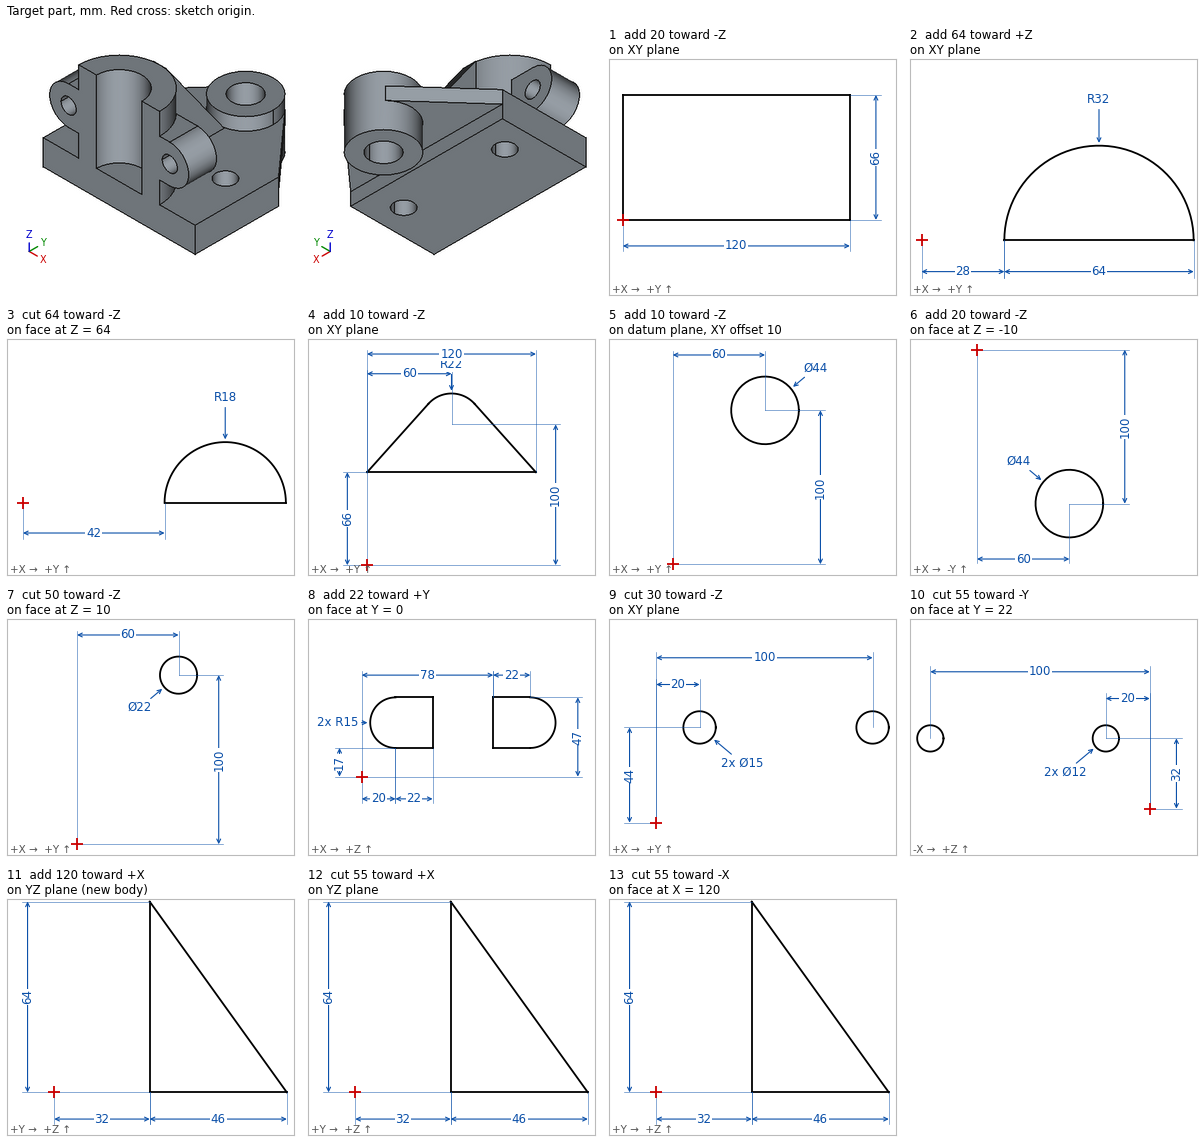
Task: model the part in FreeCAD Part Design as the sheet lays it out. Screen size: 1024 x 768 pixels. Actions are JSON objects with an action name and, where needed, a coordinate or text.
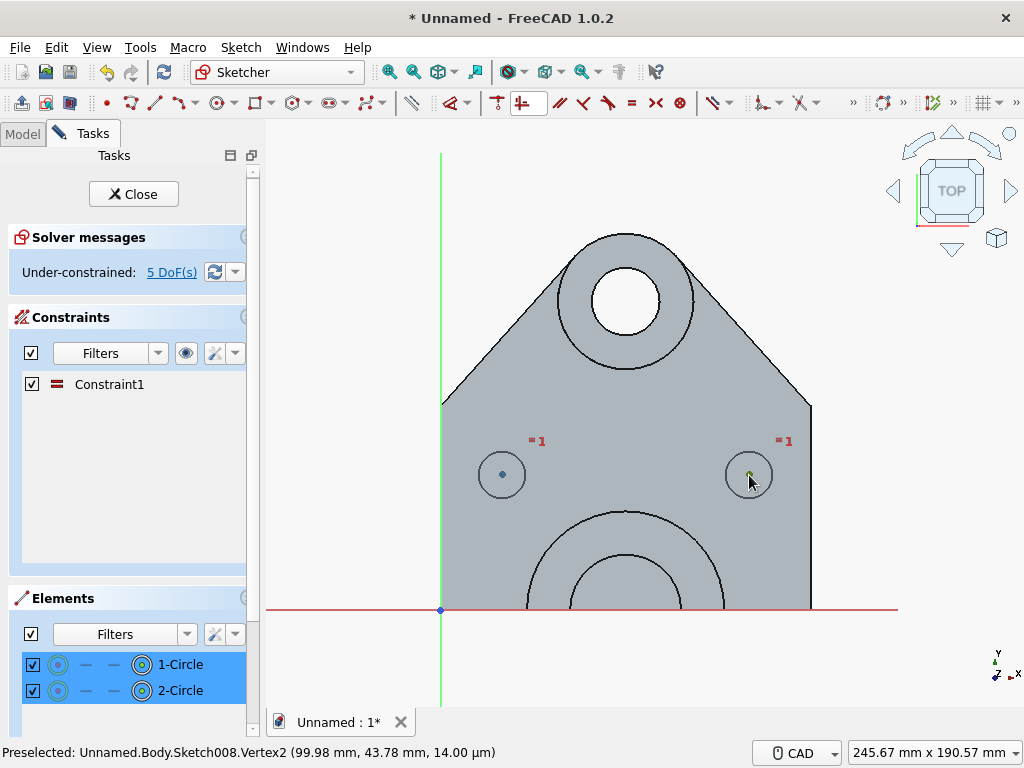
{"action": "key", "text": "h"}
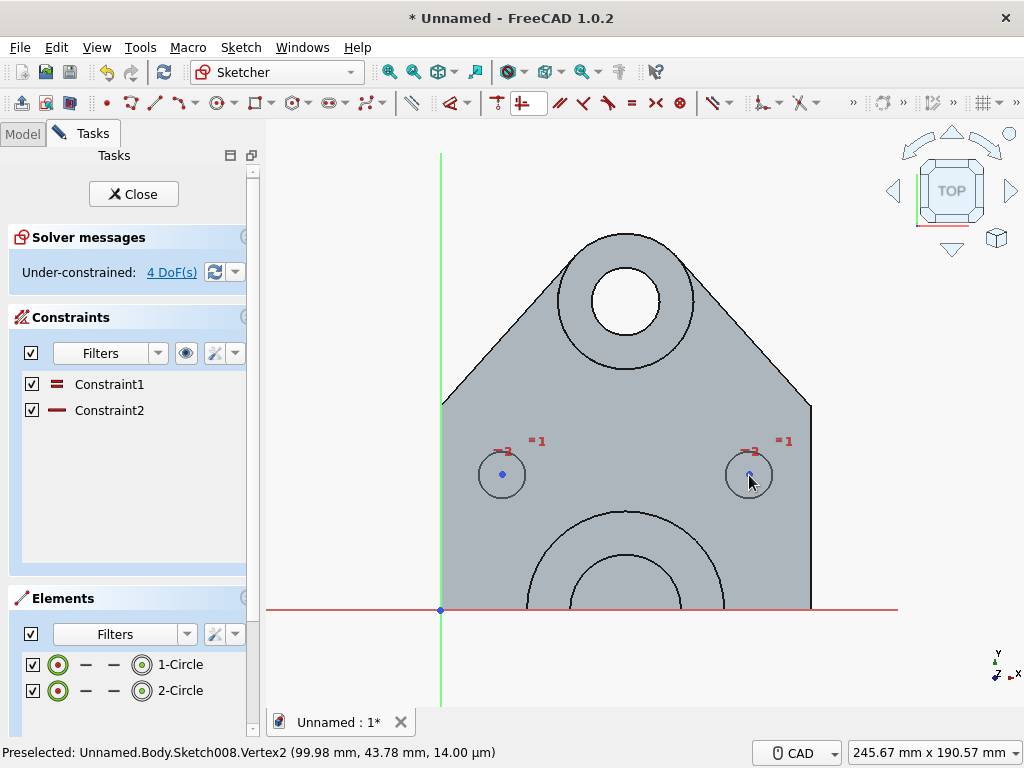
{"action": "left_click", "coordinate": [450, 104]}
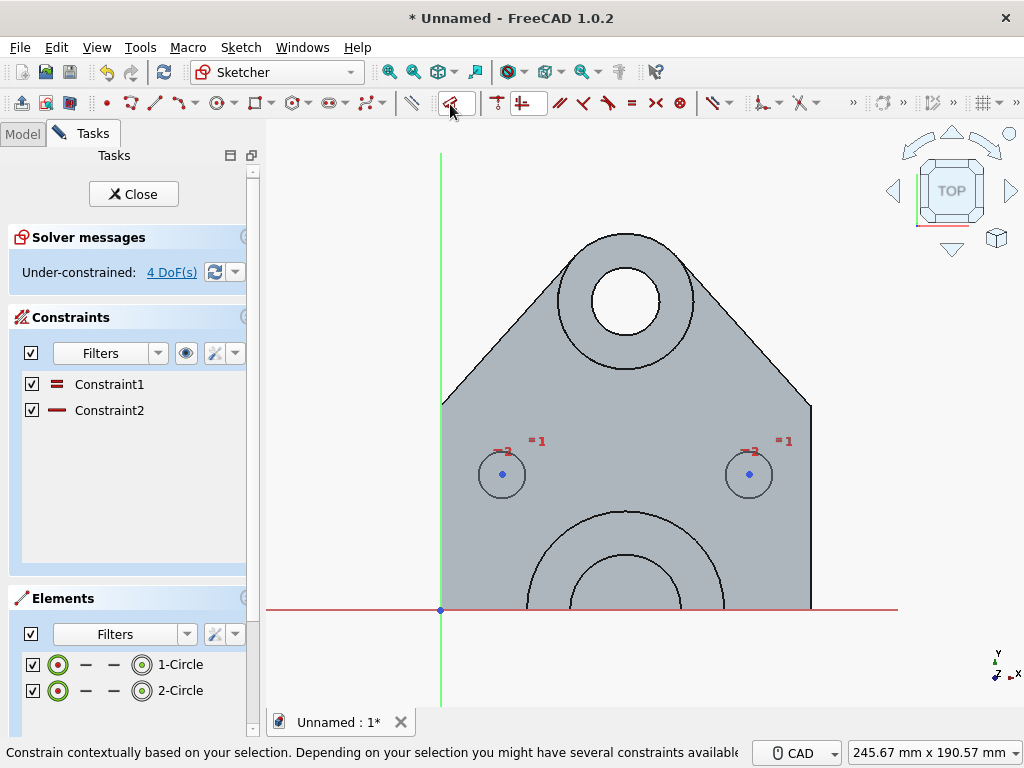
{"action": "left_click", "coordinate": [518, 458]}
{"action": "left_click", "coordinate": [540, 435]}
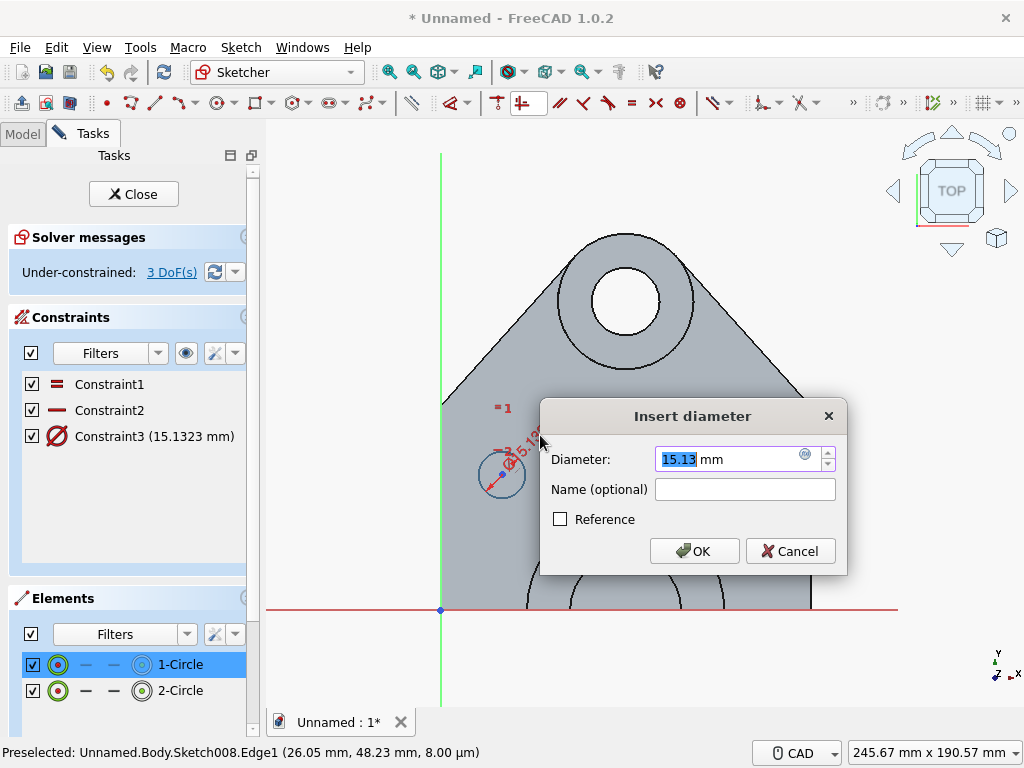
{"action": "type", "text": "15"}
{"action": "key", "text": "Return"}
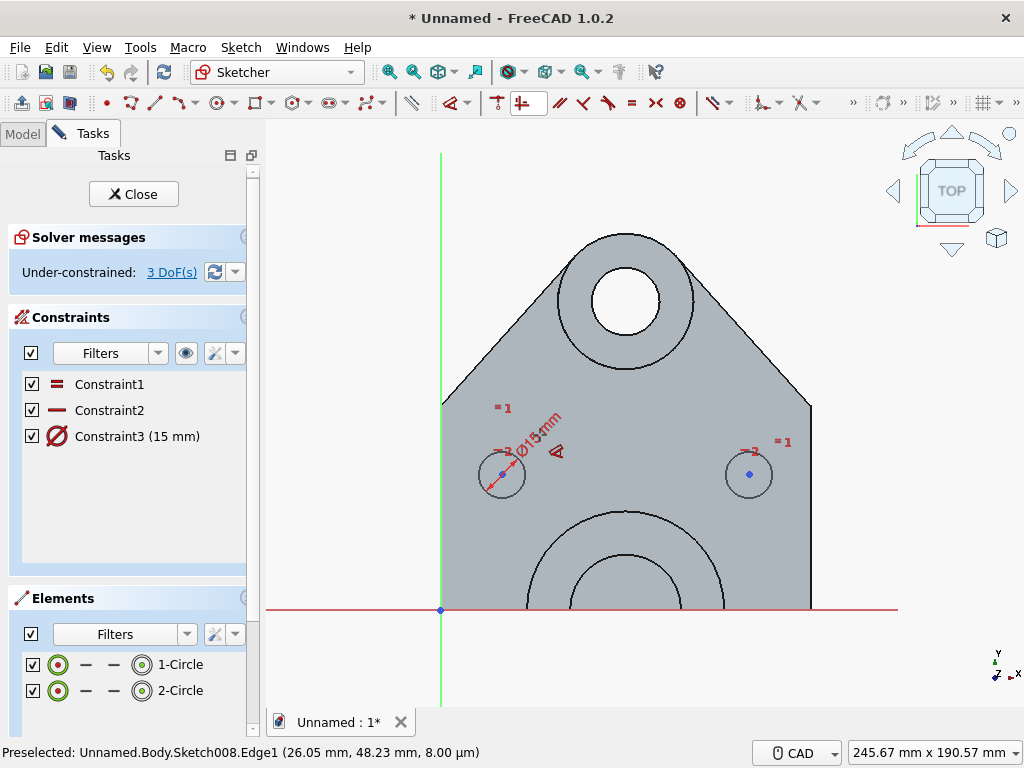
{"action": "left_click", "coordinate": [502, 475]}
{"action": "left_click", "coordinate": [471, 644]}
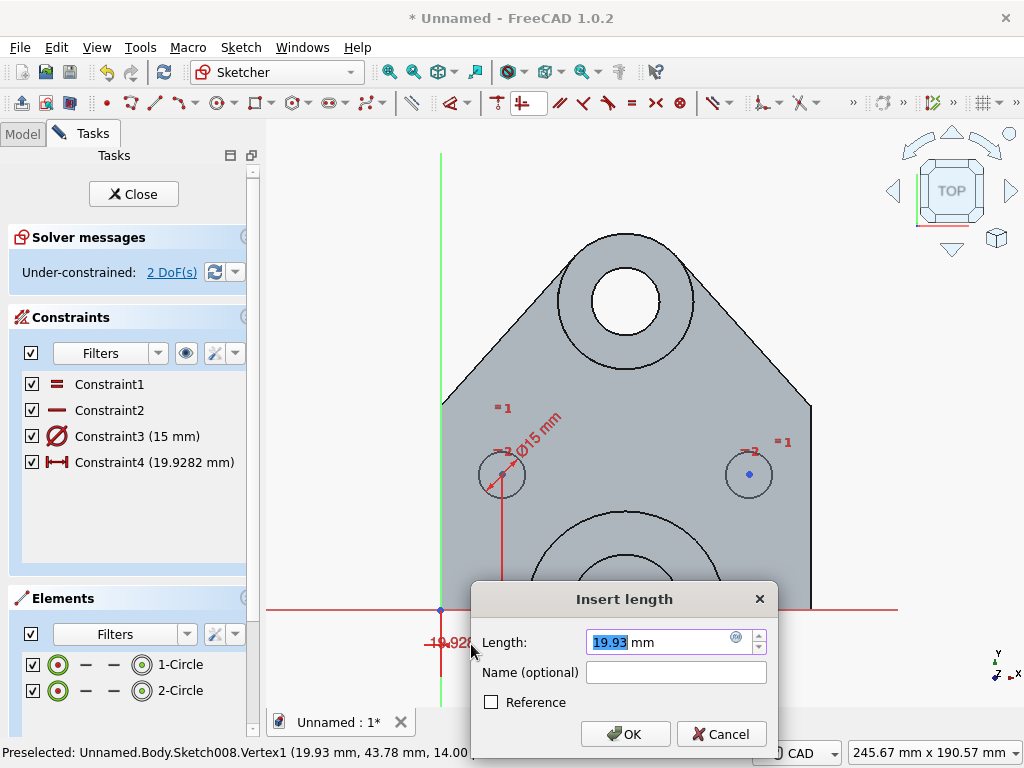
{"action": "type", "text": "20"}
{"action": "key", "text": "Return"}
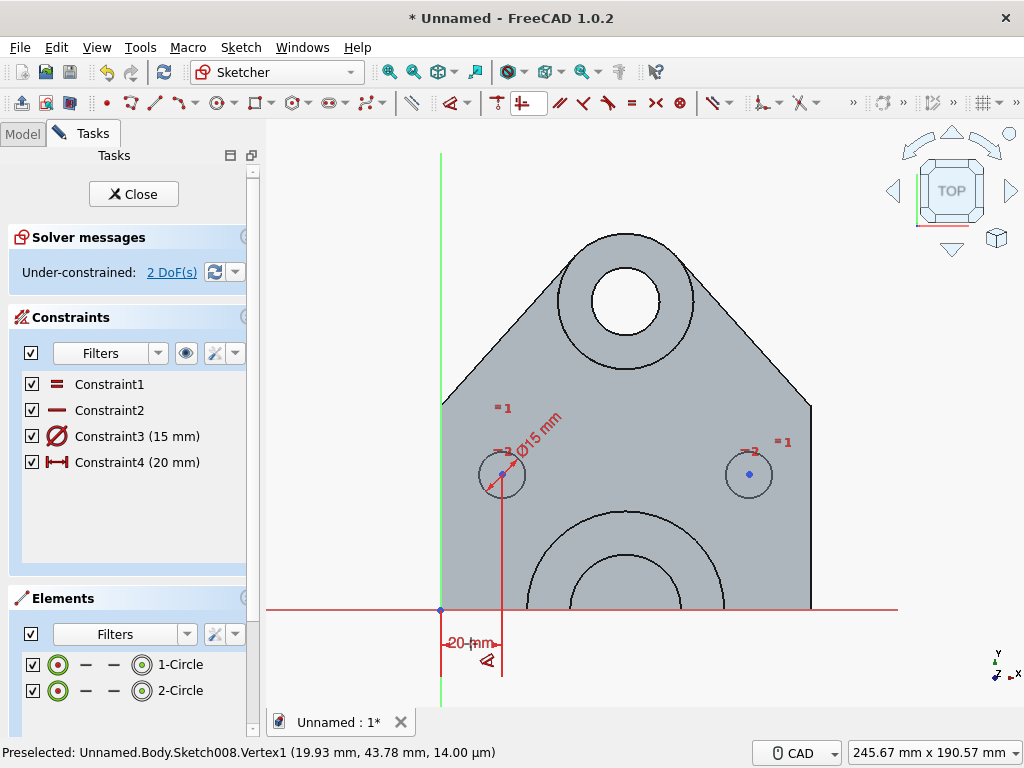
{"action": "left_click", "coordinate": [502, 475]}
{"action": "left_click", "coordinate": [407, 543]}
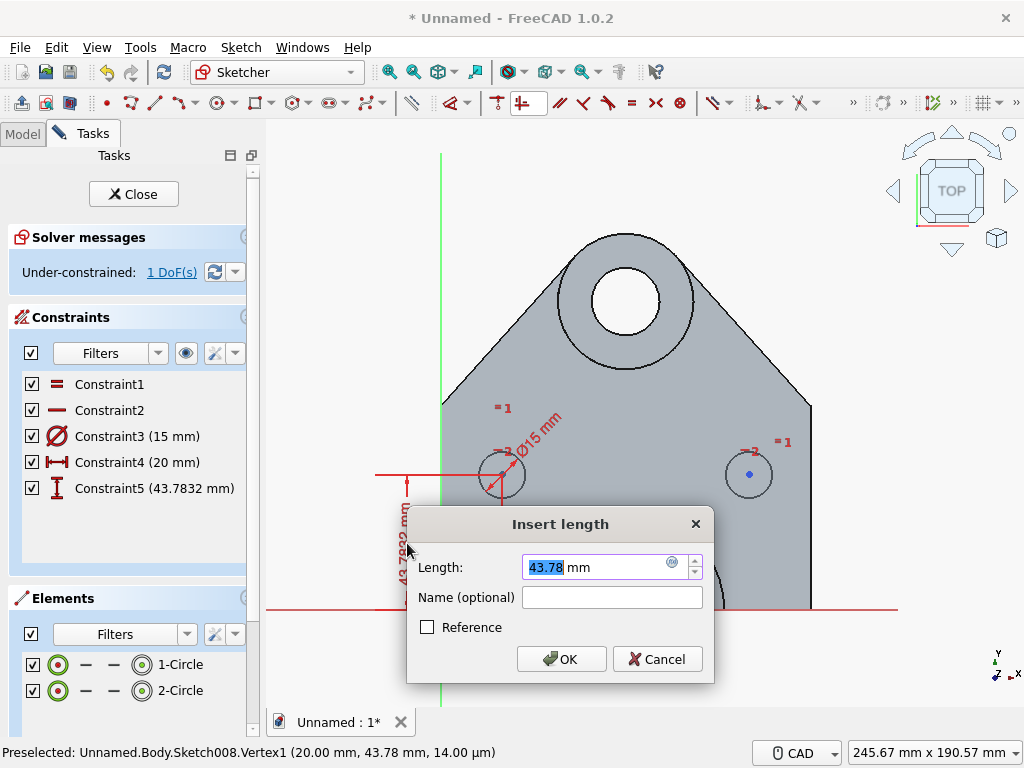
{"action": "type", "text": "44"}
{"action": "key", "text": "Return"}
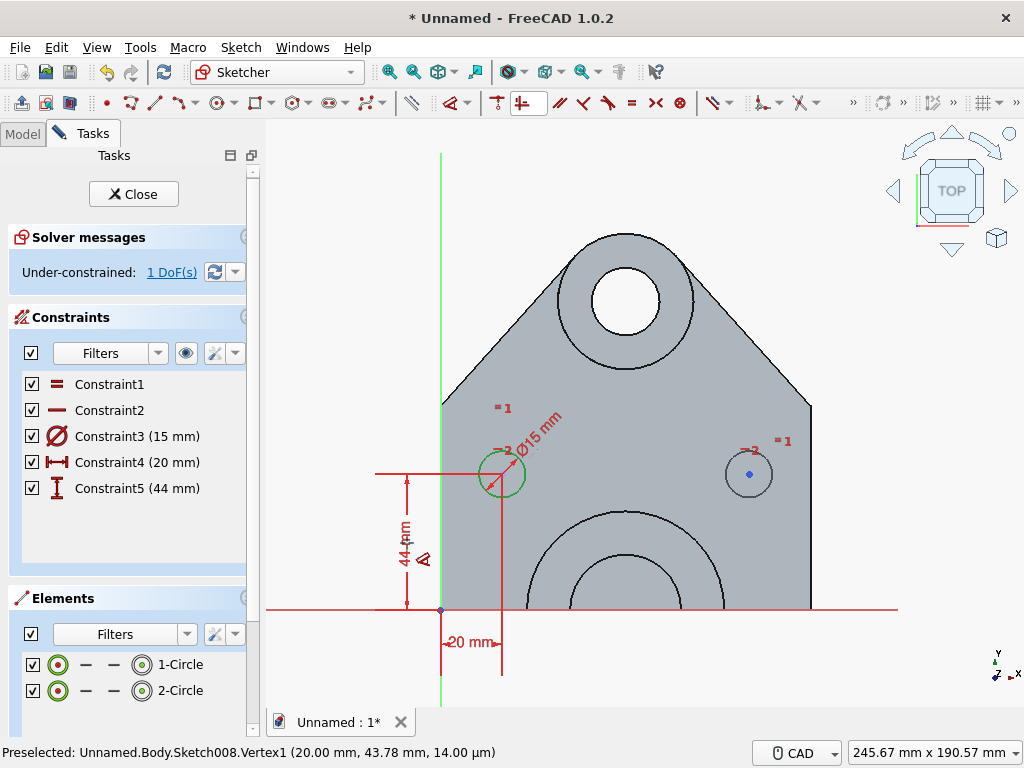
{"action": "left_click", "coordinate": [749, 474]}
{"action": "left_click", "coordinate": [595, 644]}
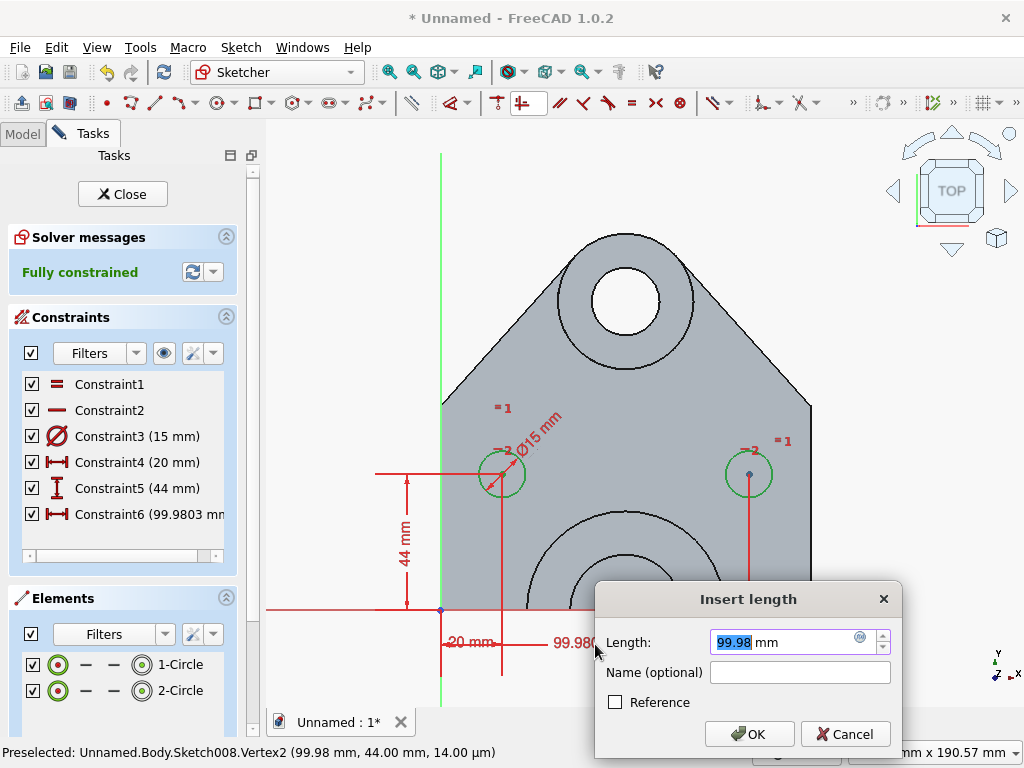
{"action": "type", "text": "100"}
{"action": "key", "text": "Return"}
{"action": "key", "text": "Escape"}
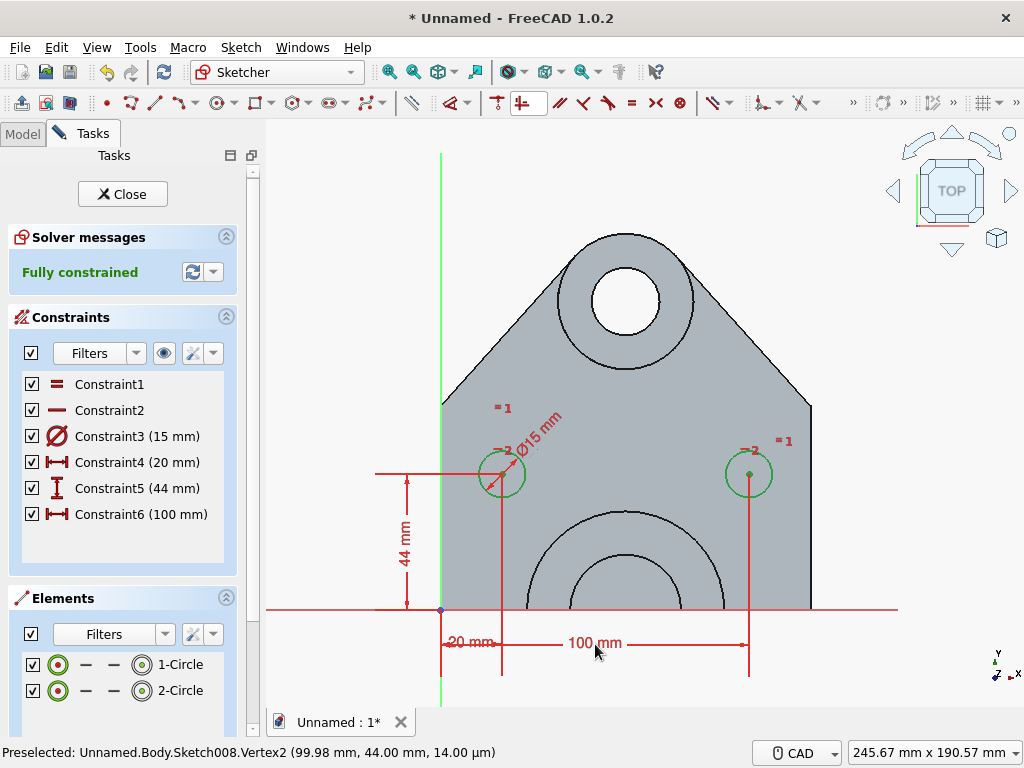
{"action": "left_click", "coordinate": [123, 194]}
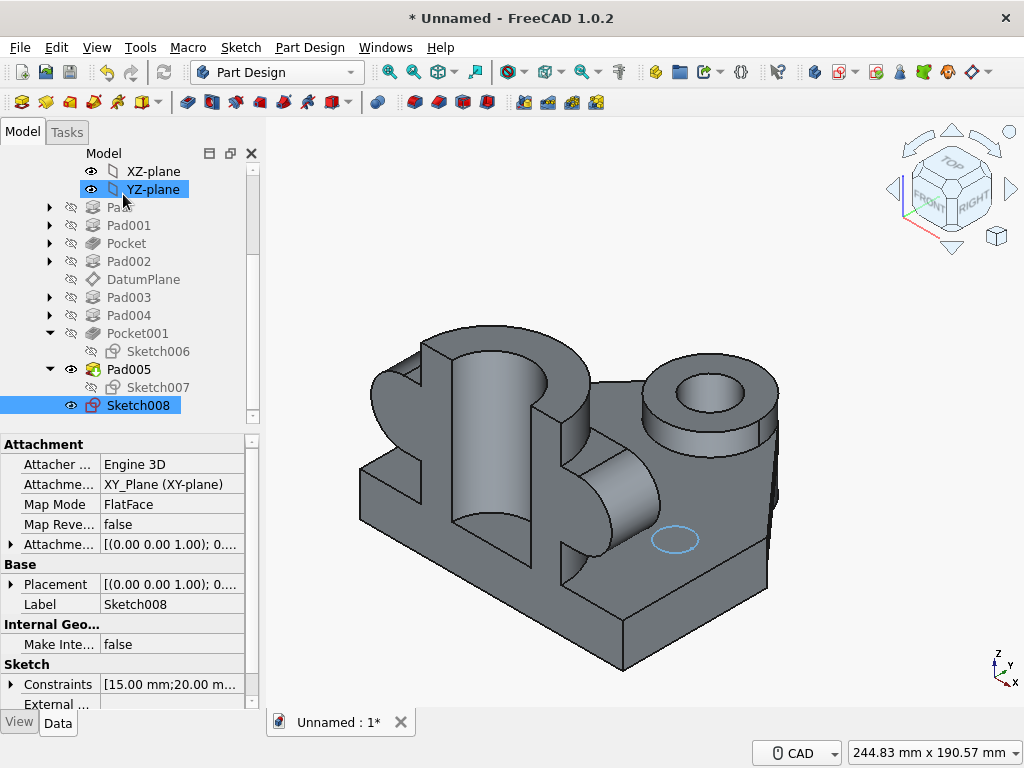
{"action": "left_click", "coordinate": [188, 102]}